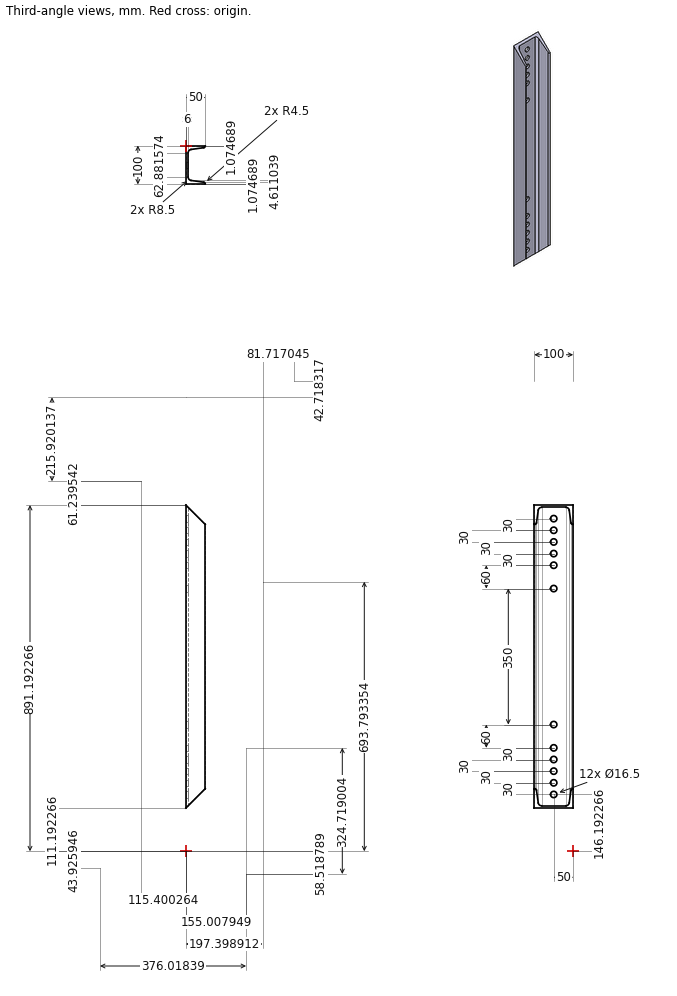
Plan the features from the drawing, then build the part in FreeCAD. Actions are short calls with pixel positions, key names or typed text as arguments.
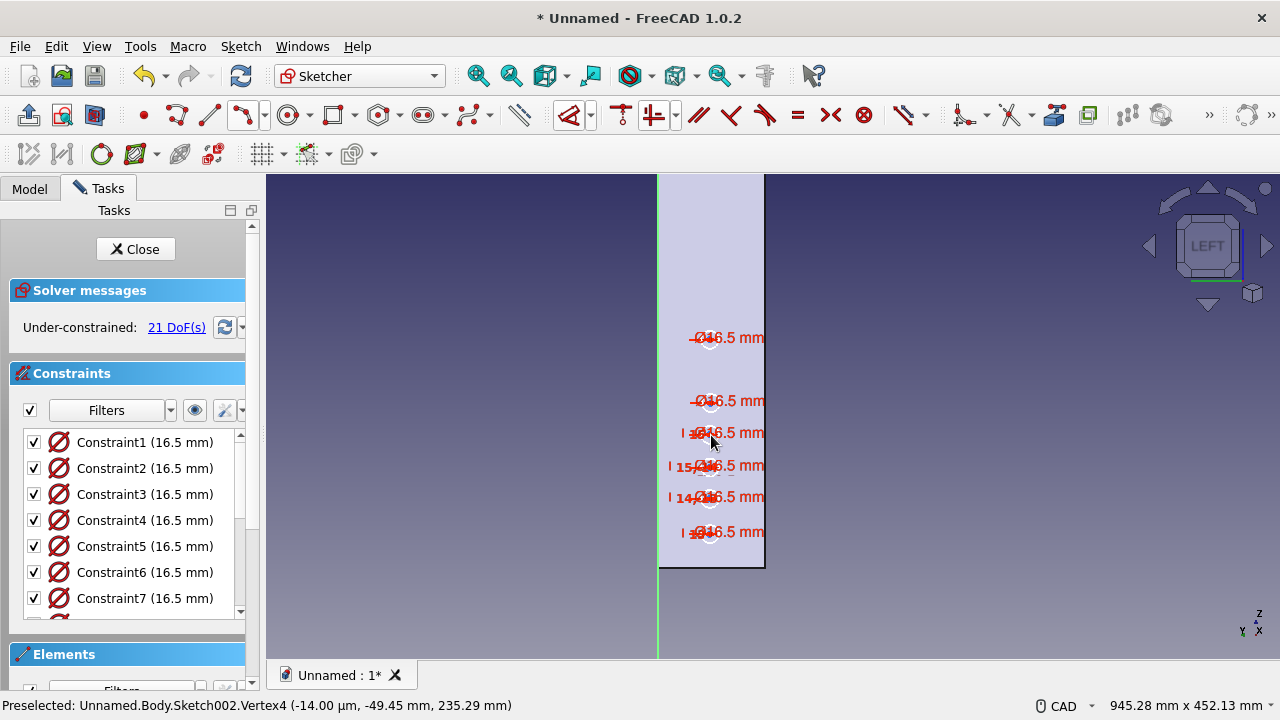
click(710, 435)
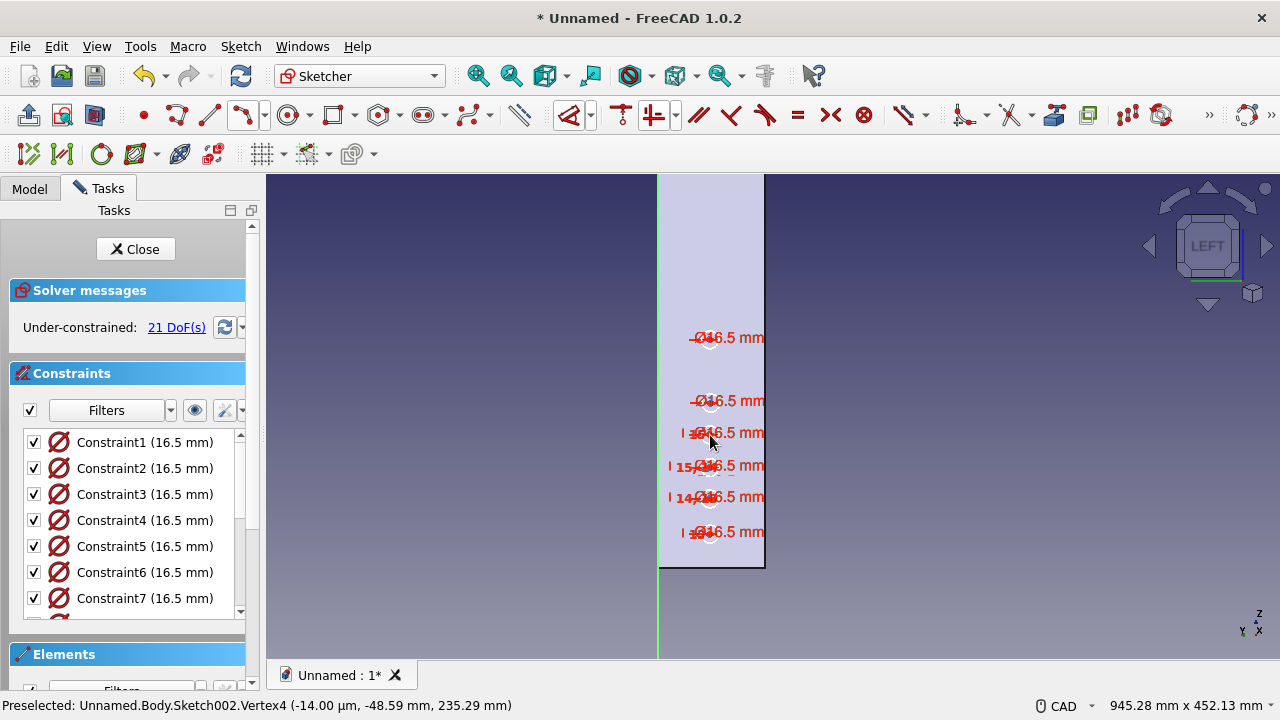
click(711, 403)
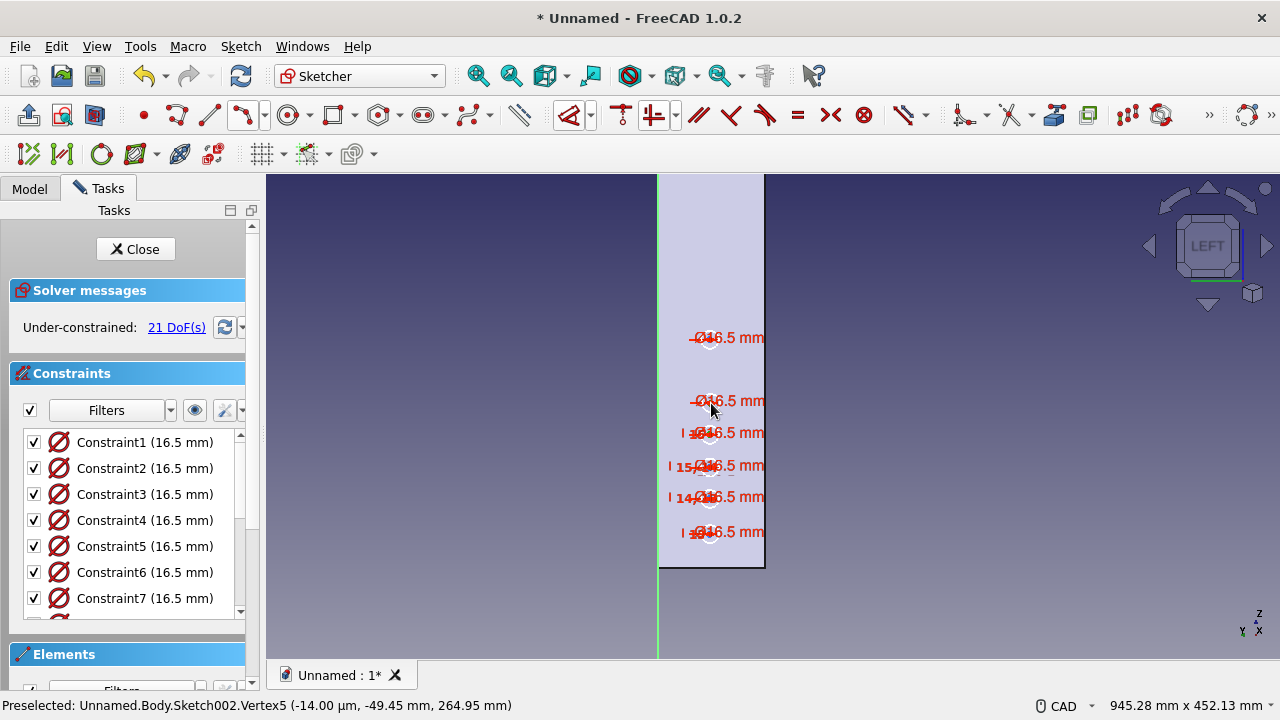
click(676, 116)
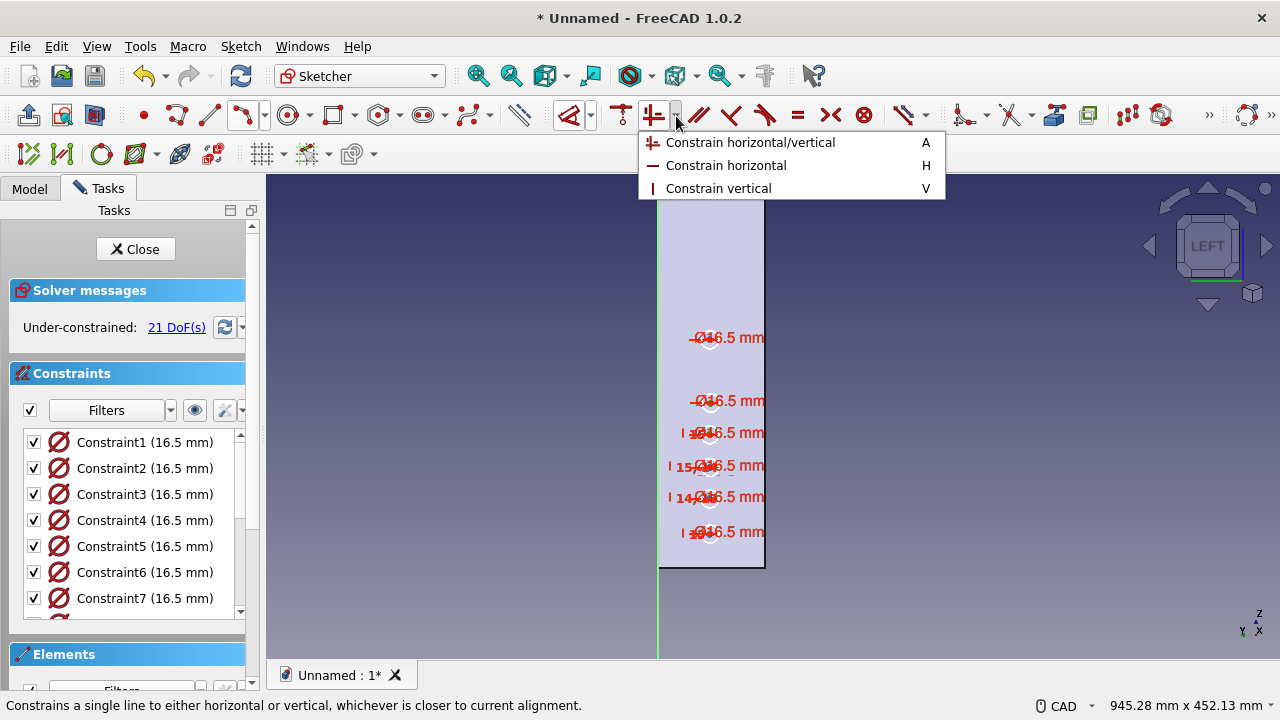
click(792, 188)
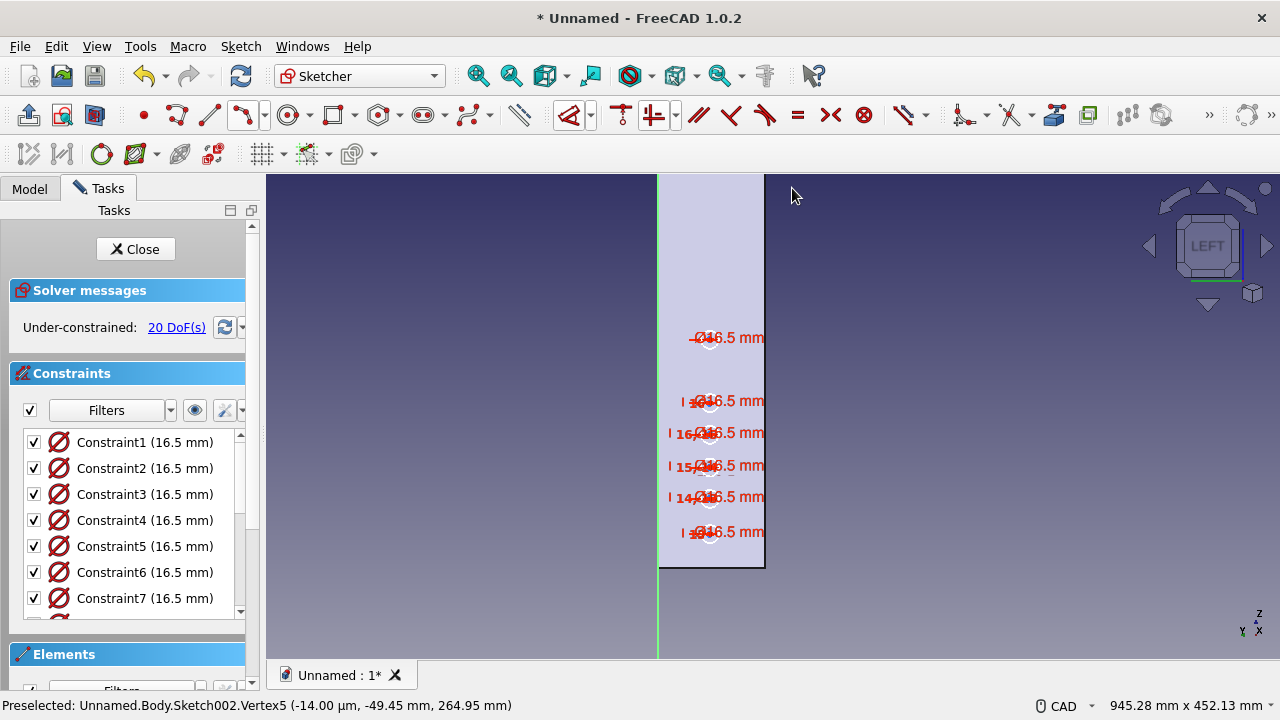
click(710, 403)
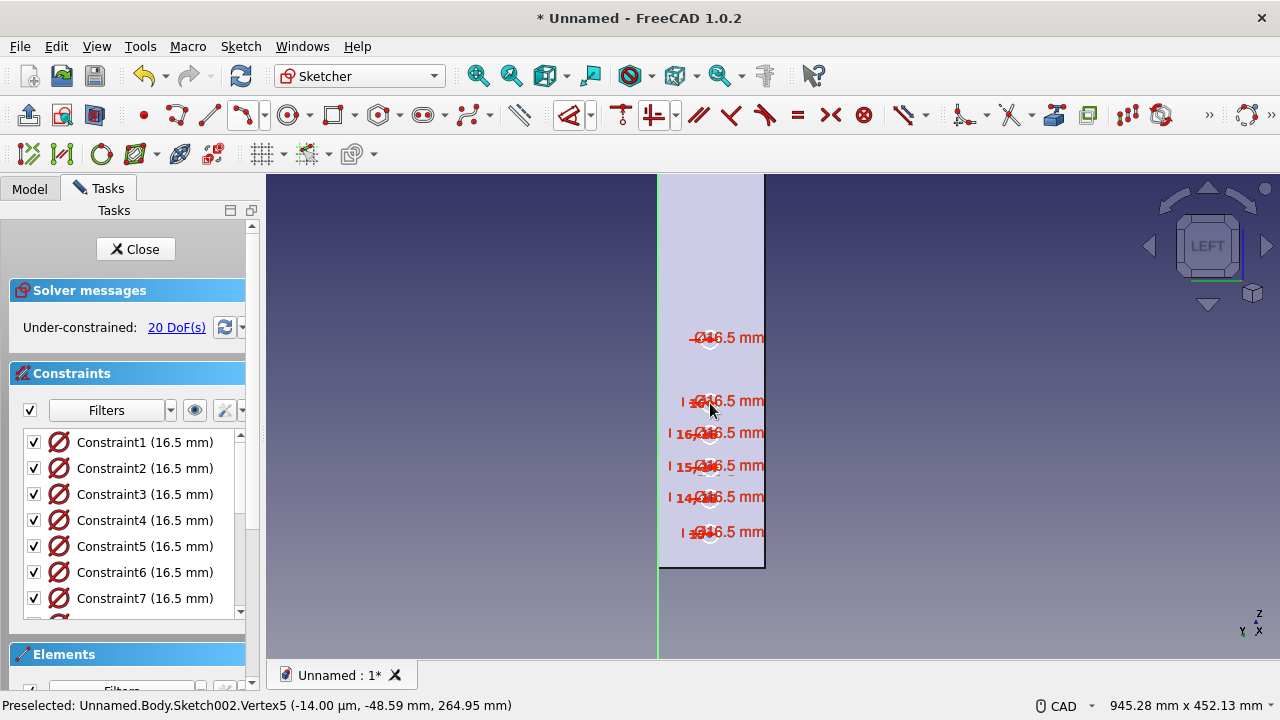
click(710, 340)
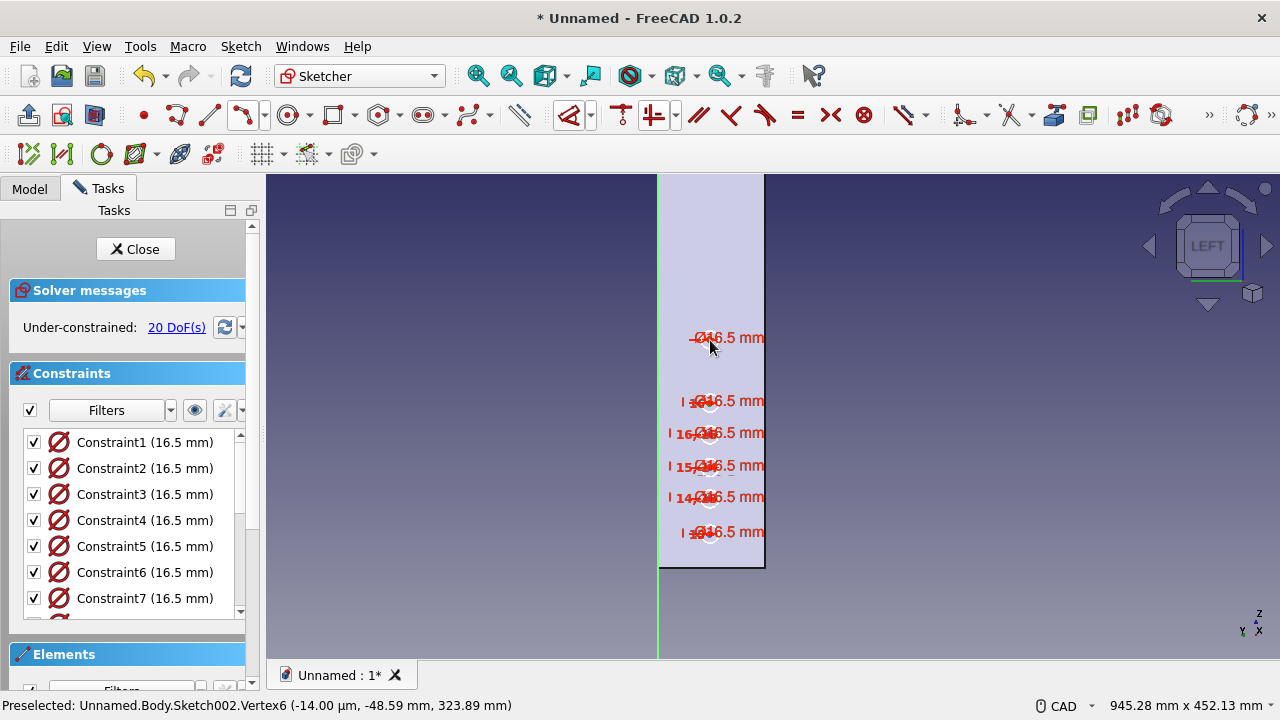
click(676, 116)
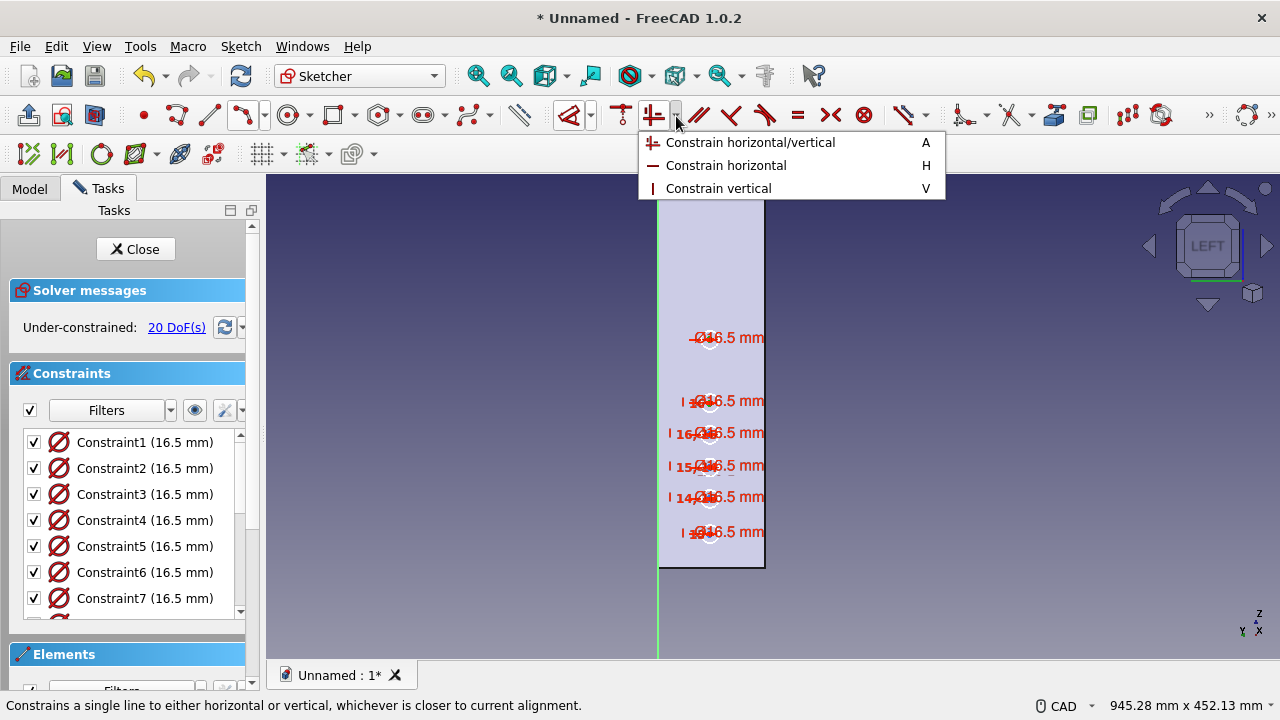
click(792, 188)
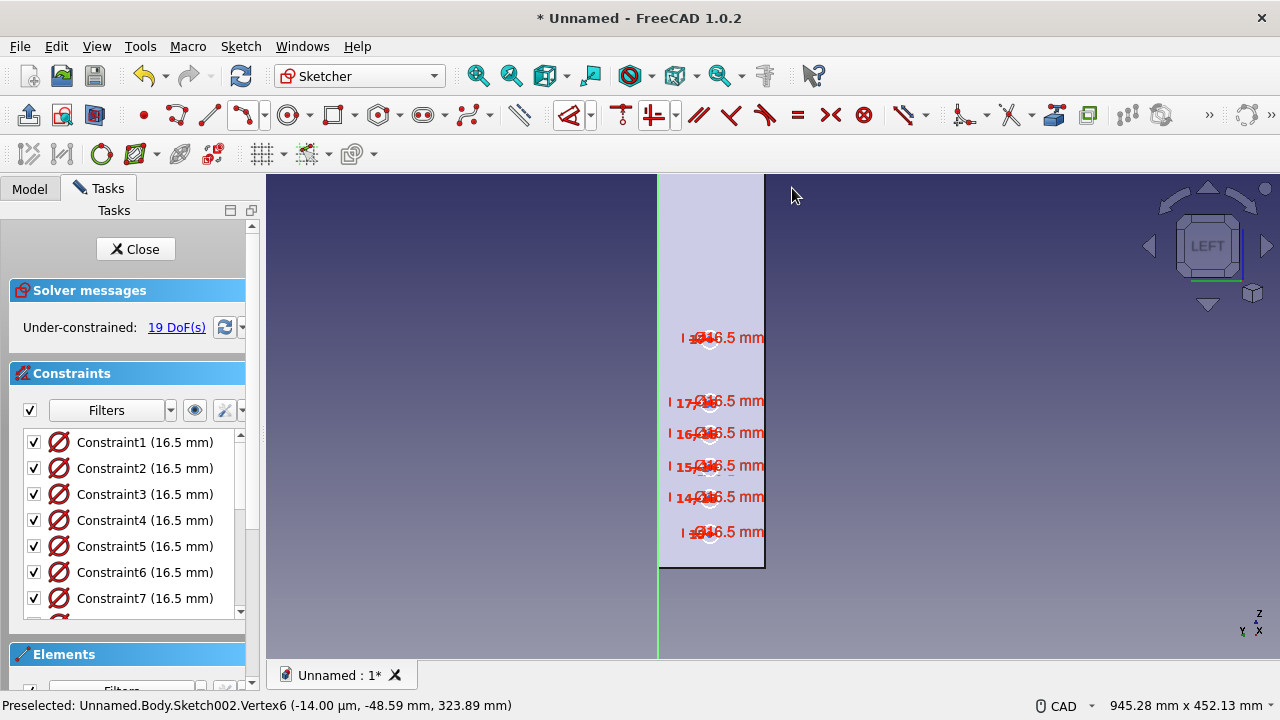
click(710, 340)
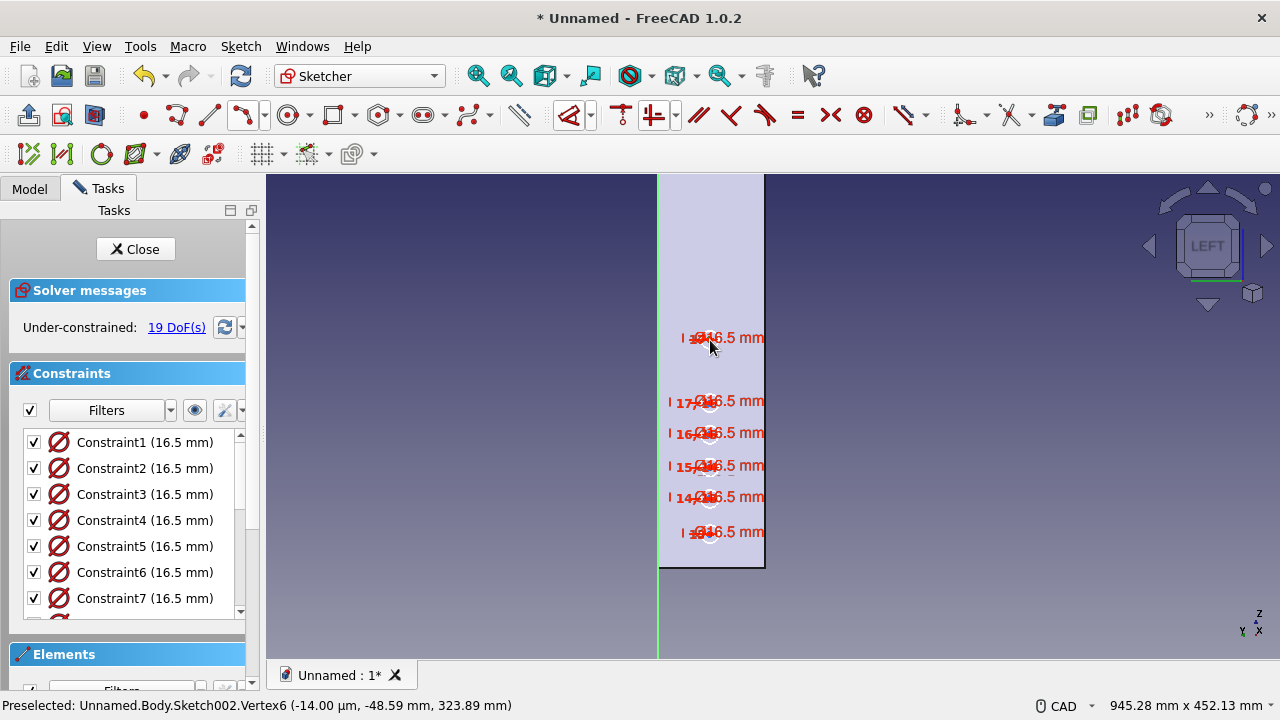
scroll(711, 500, down, 6)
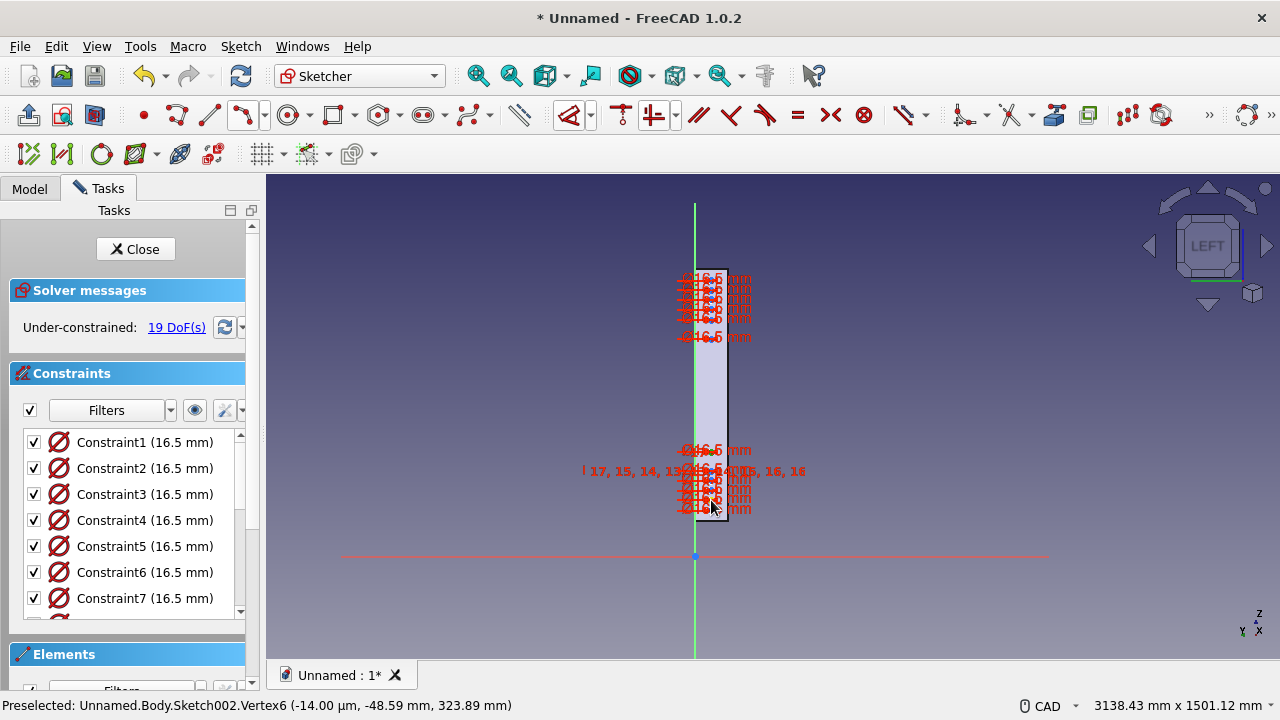
click(711, 339)